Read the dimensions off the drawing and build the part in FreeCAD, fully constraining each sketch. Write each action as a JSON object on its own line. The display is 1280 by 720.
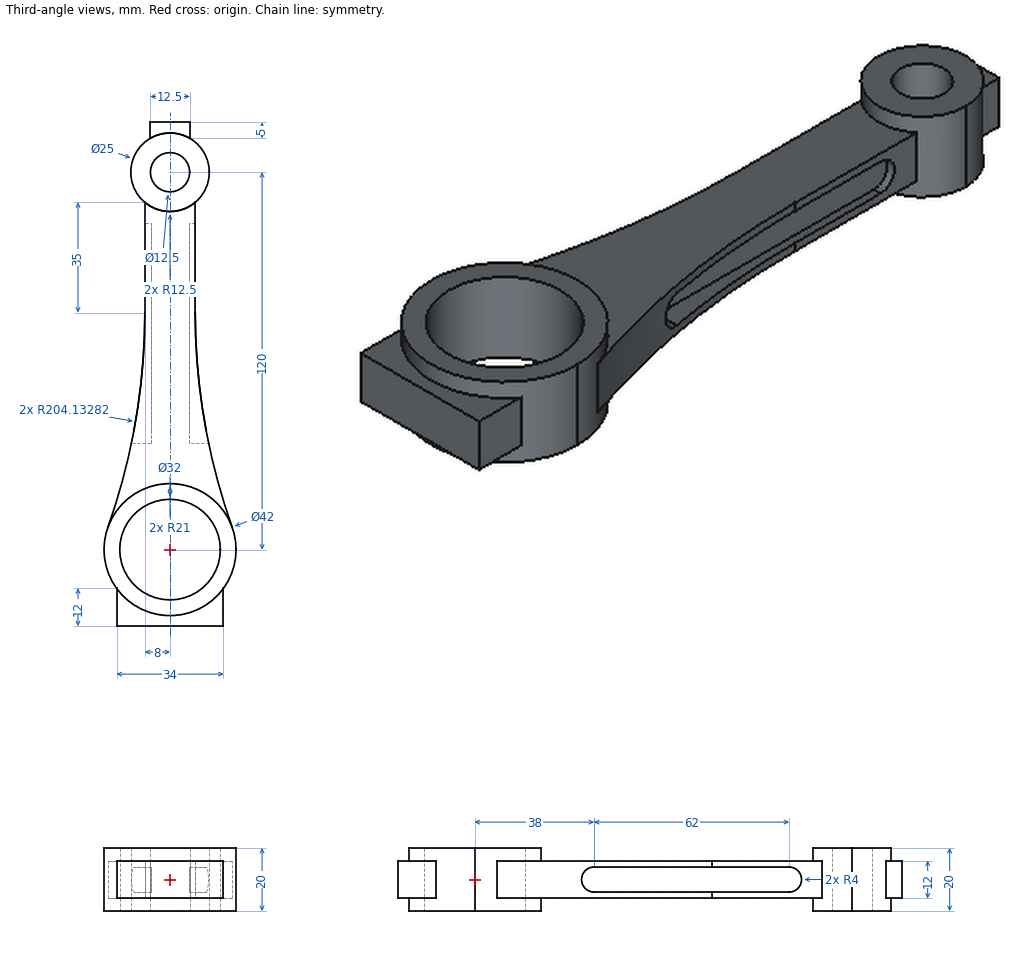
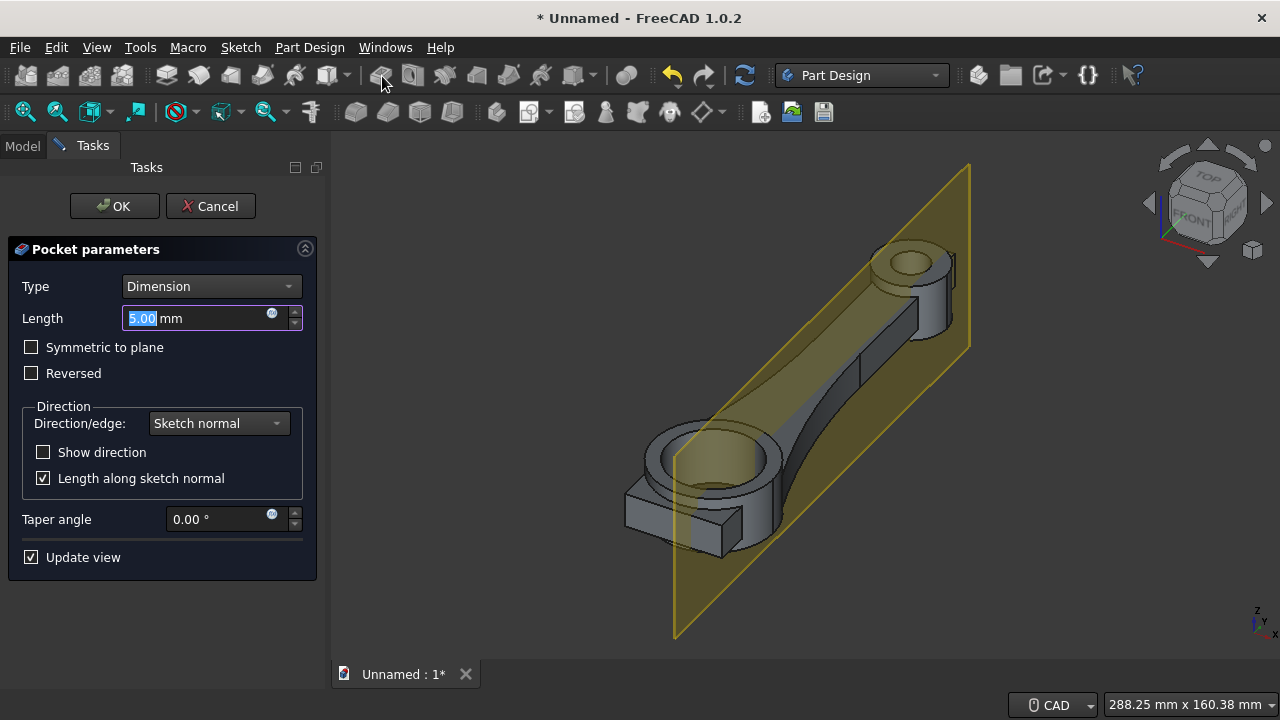
{"action": "left_click", "coordinate": [212, 286]}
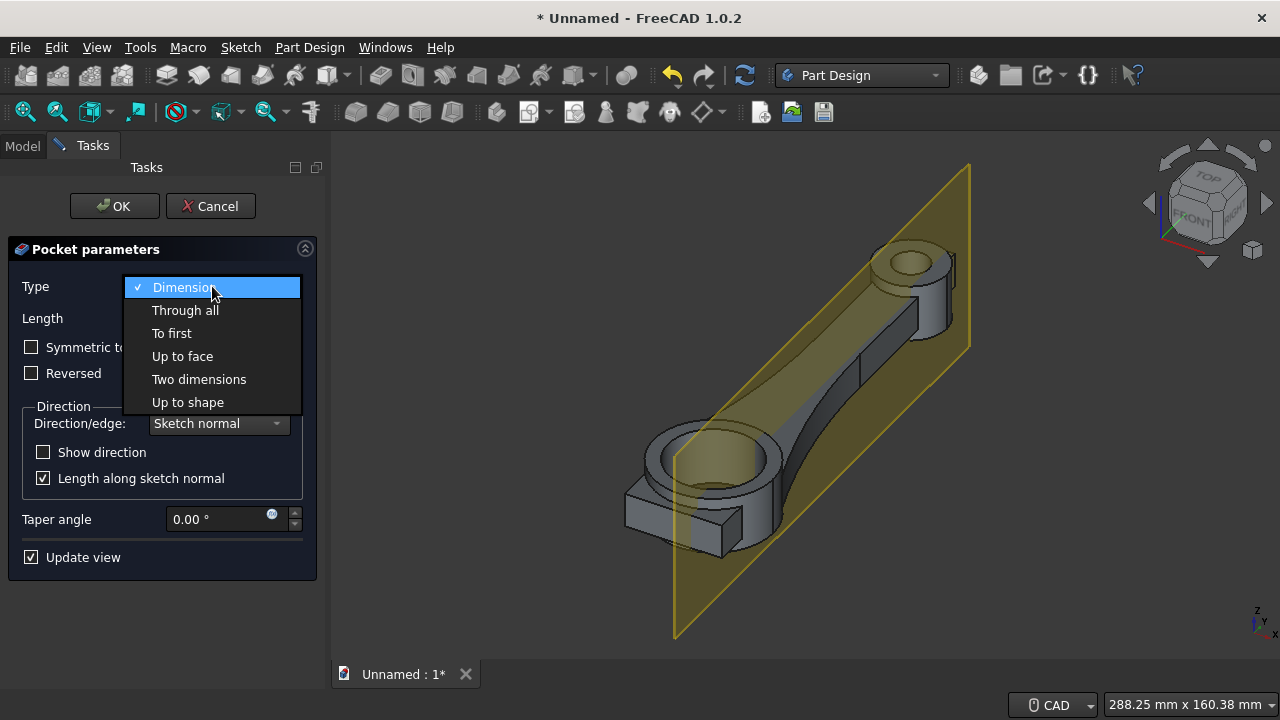
{"action": "left_click", "coordinate": [212, 310]}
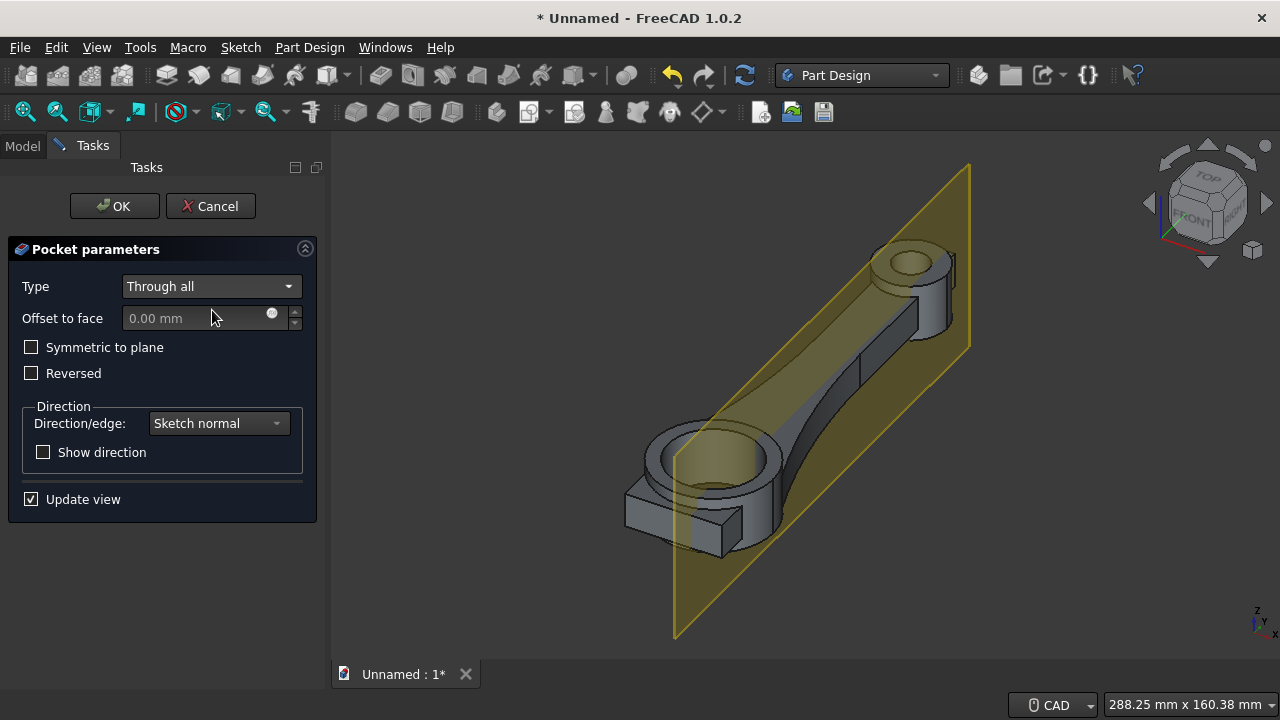
{"action": "left_click", "coordinate": [30, 373]}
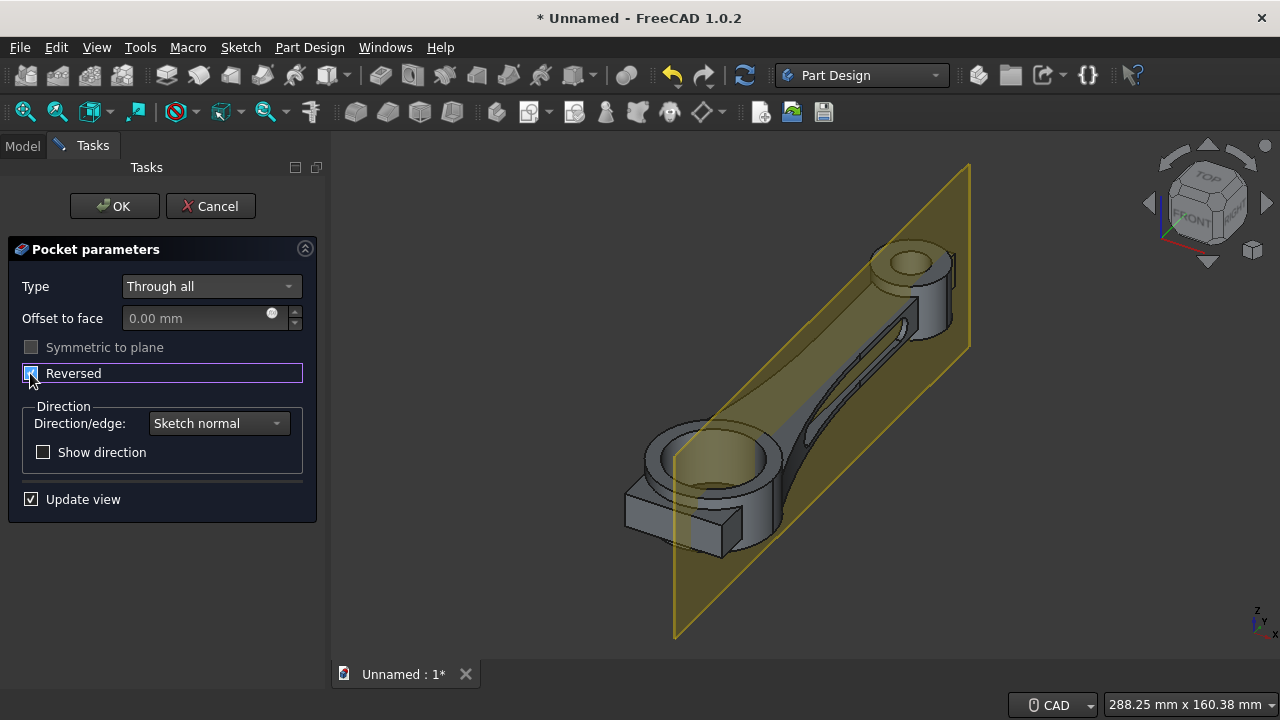
{"action": "left_click", "coordinate": [115, 206]}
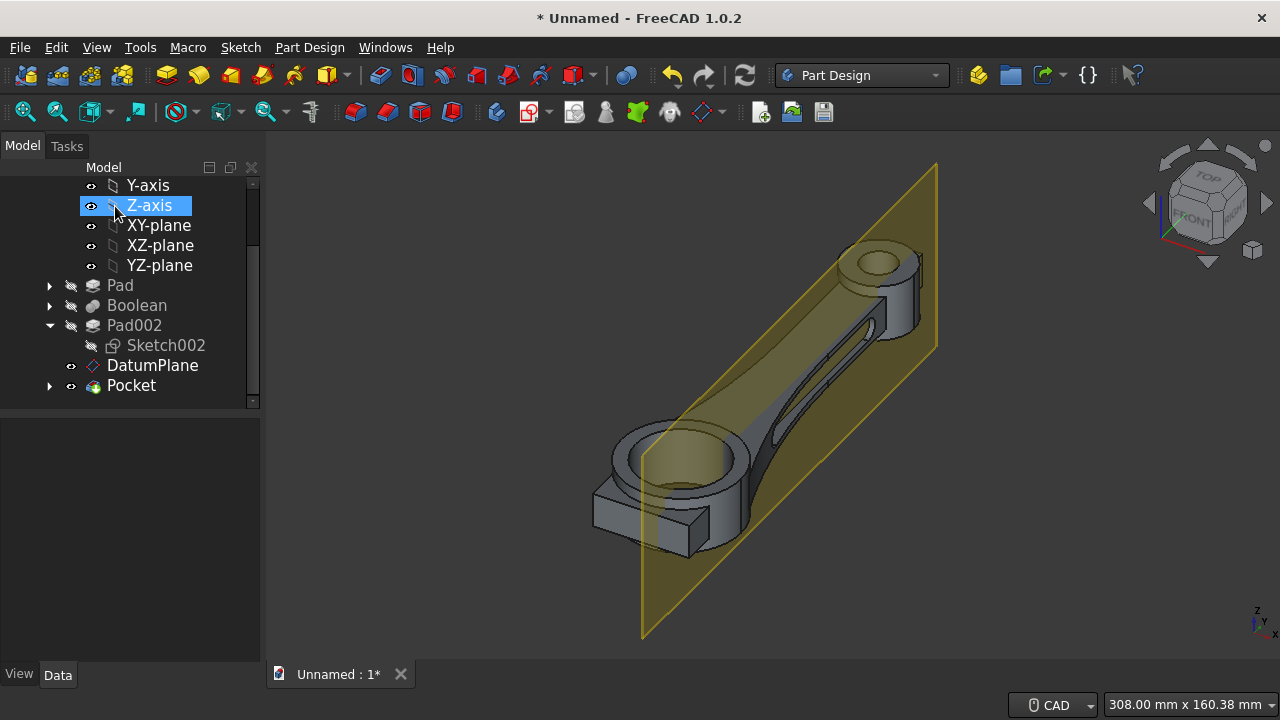
{"action": "left_click", "coordinate": [116, 366]}
{"action": "key", "text": "space"}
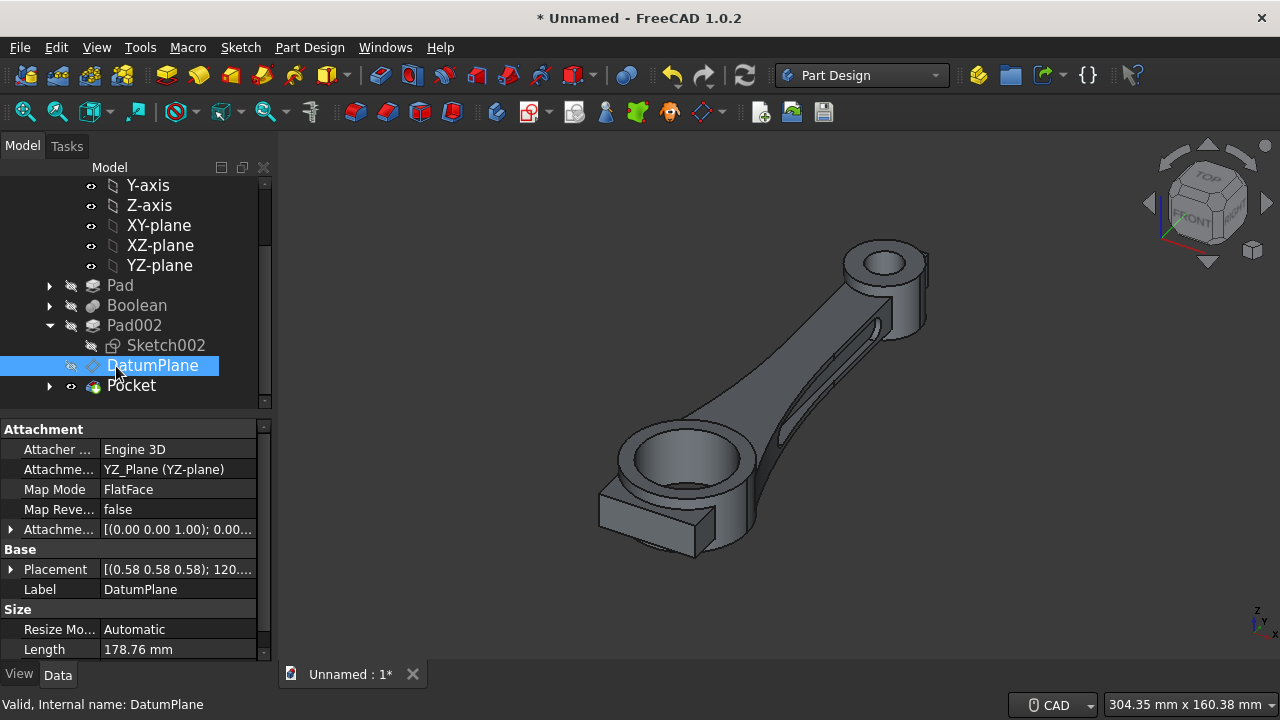
{"action": "left_click", "coordinate": [116, 386]}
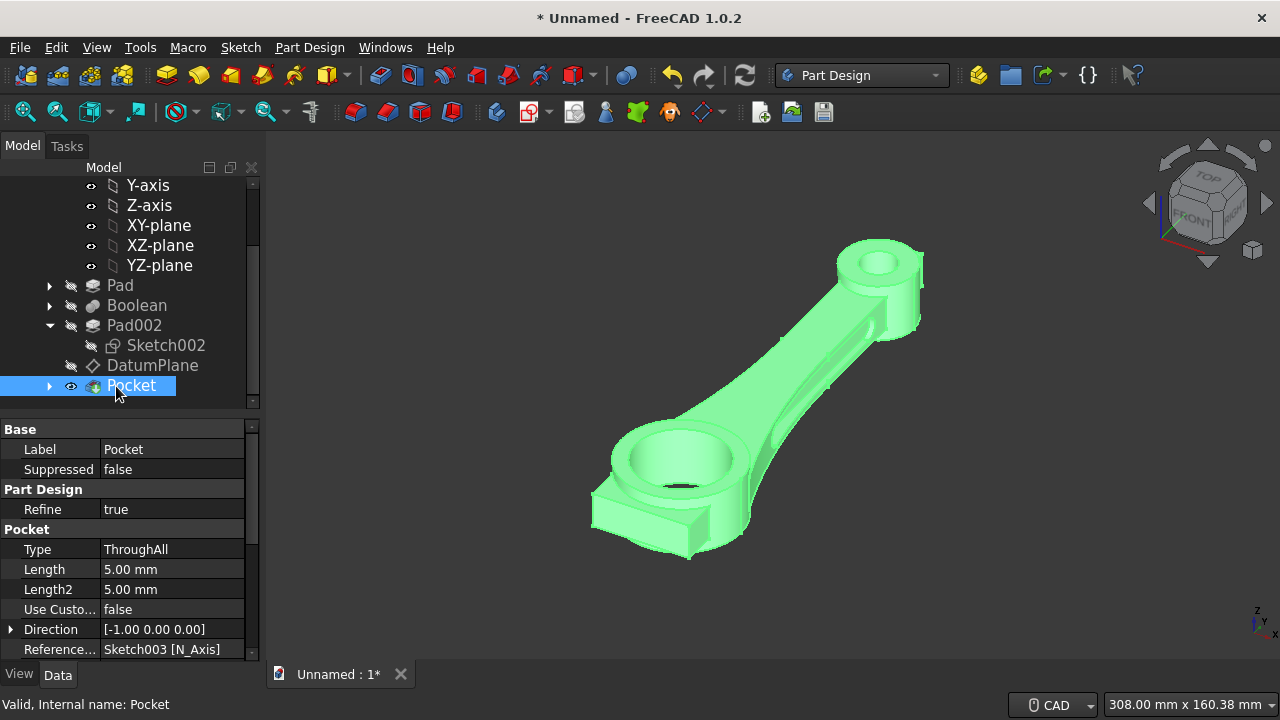
{"action": "left_click", "coordinate": [26, 76]}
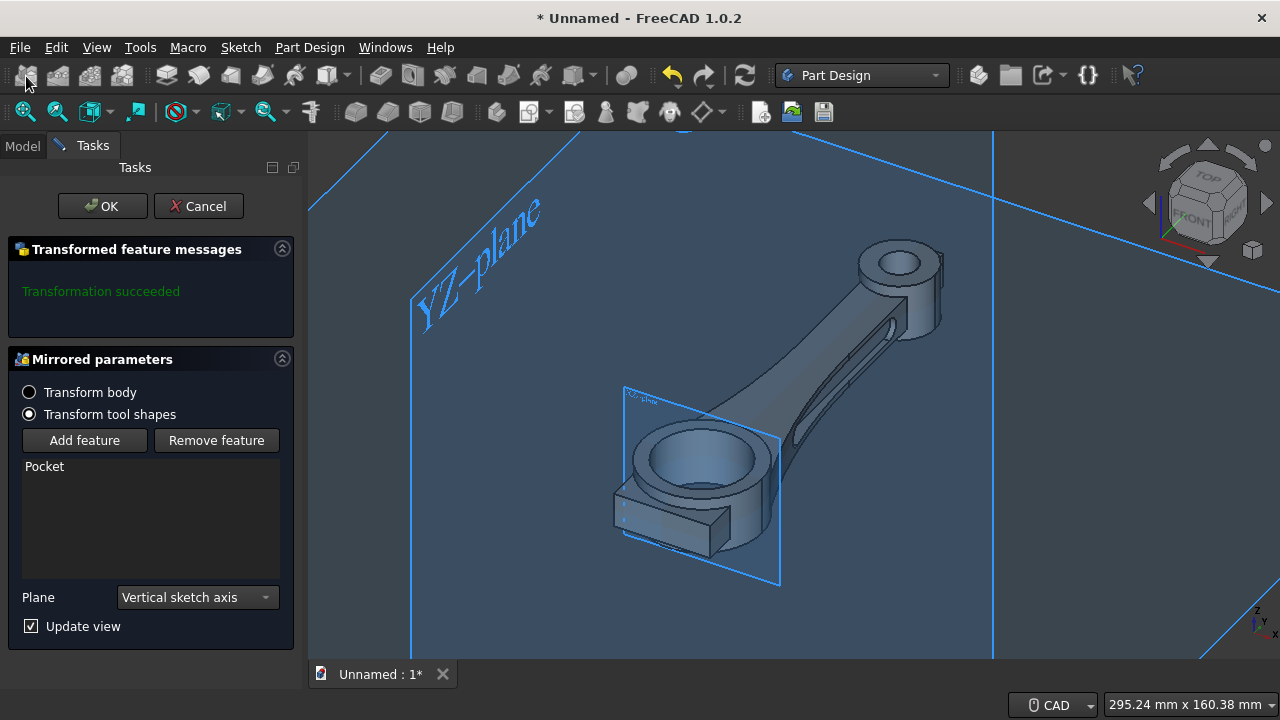
{"action": "left_click", "coordinate": [198, 598]}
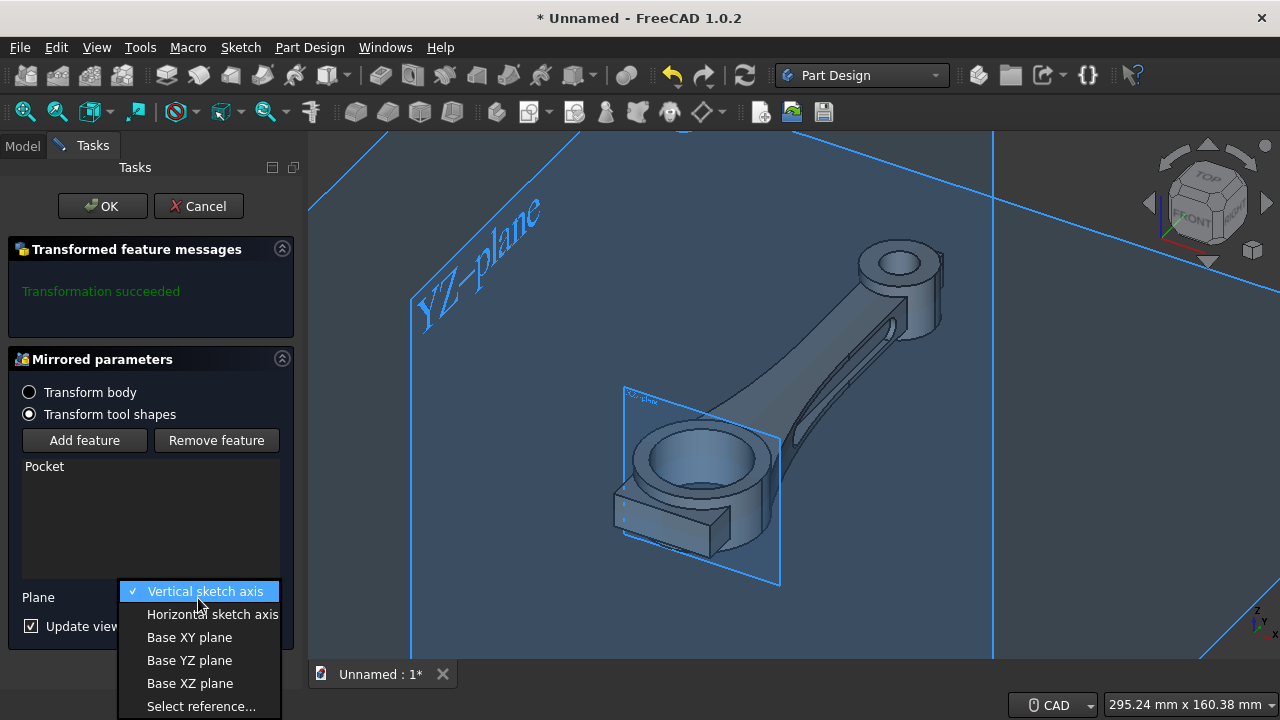
{"action": "left_click", "coordinate": [198, 660]}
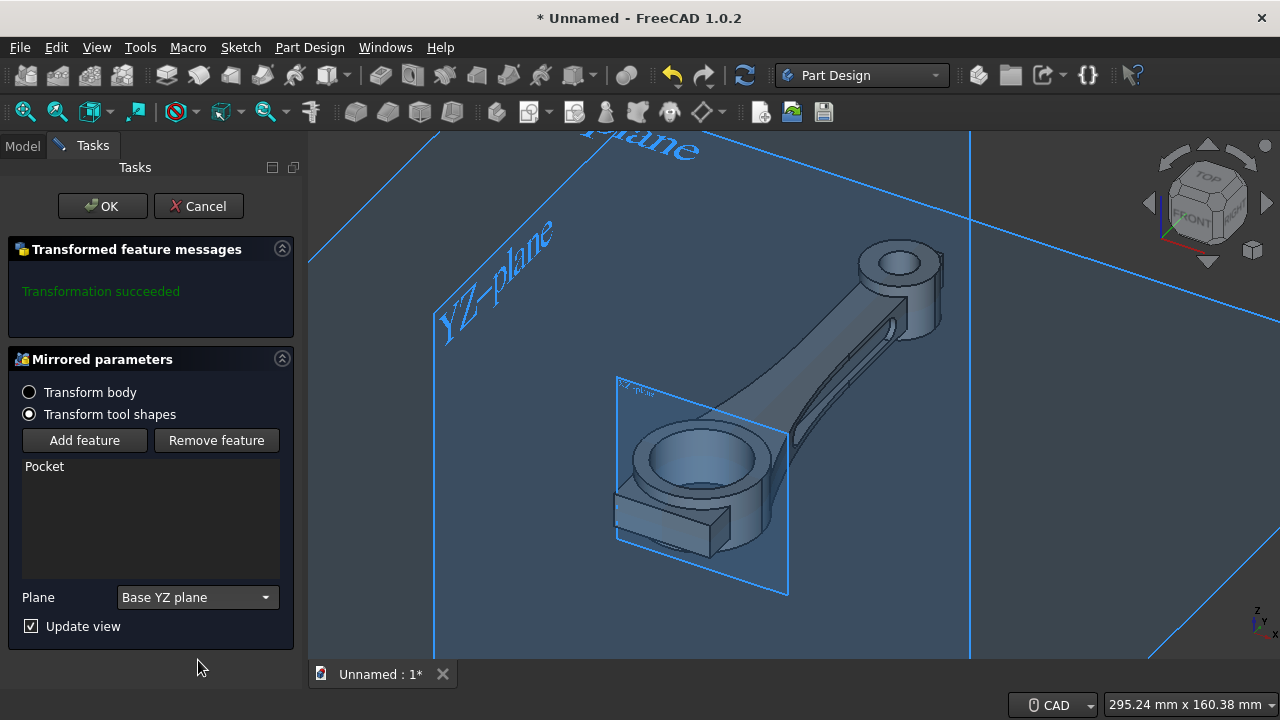
{"action": "left_click", "coordinate": [103, 206]}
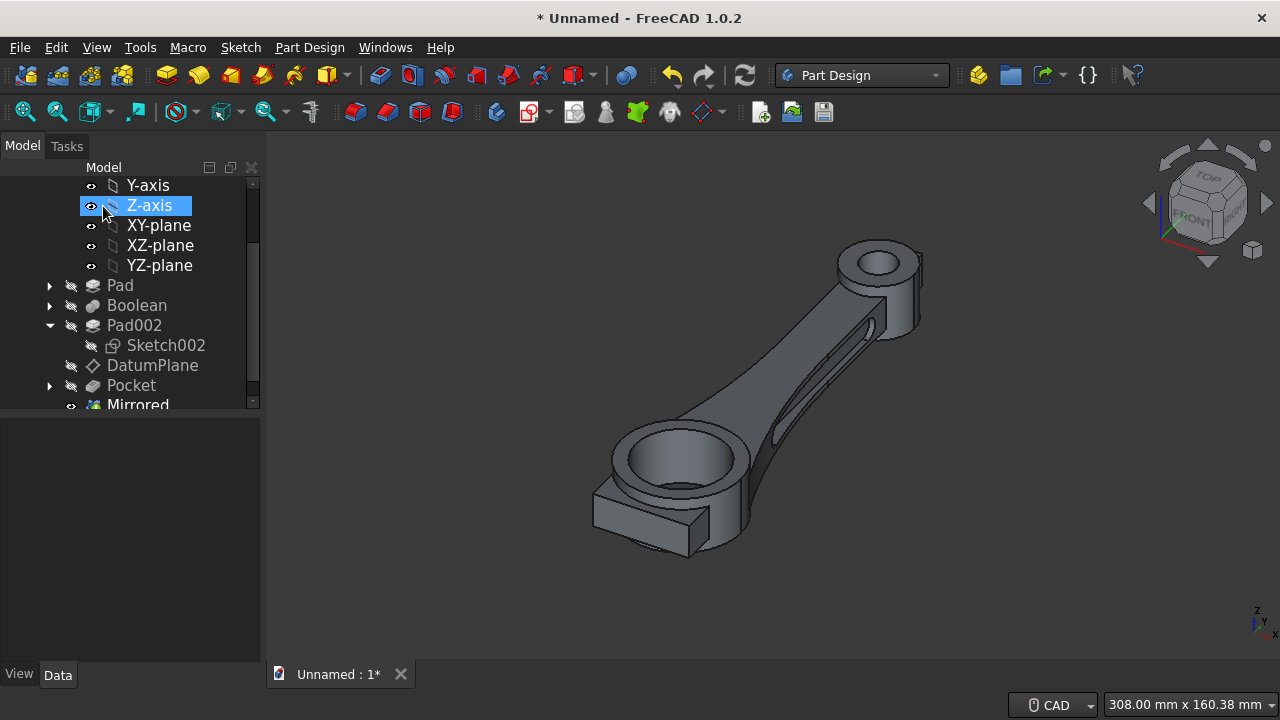
{"action": "key", "text": "0"}